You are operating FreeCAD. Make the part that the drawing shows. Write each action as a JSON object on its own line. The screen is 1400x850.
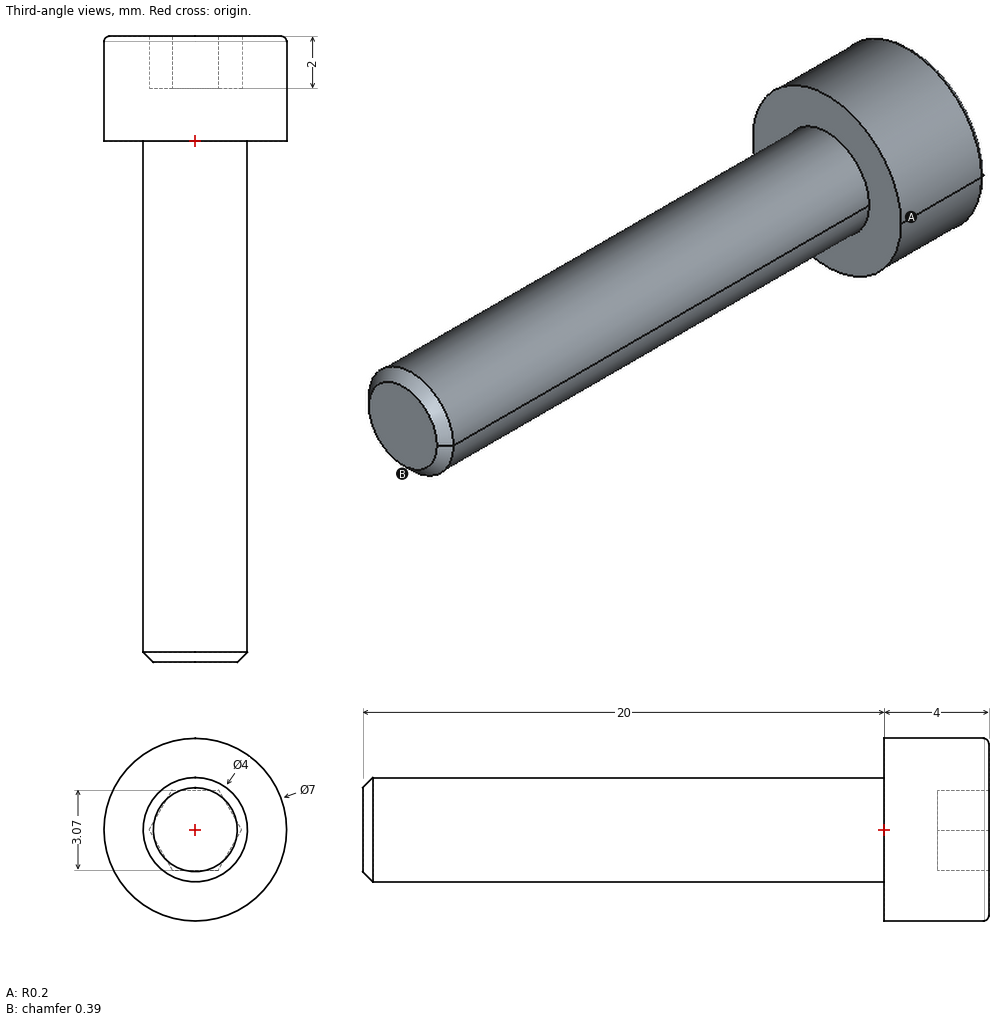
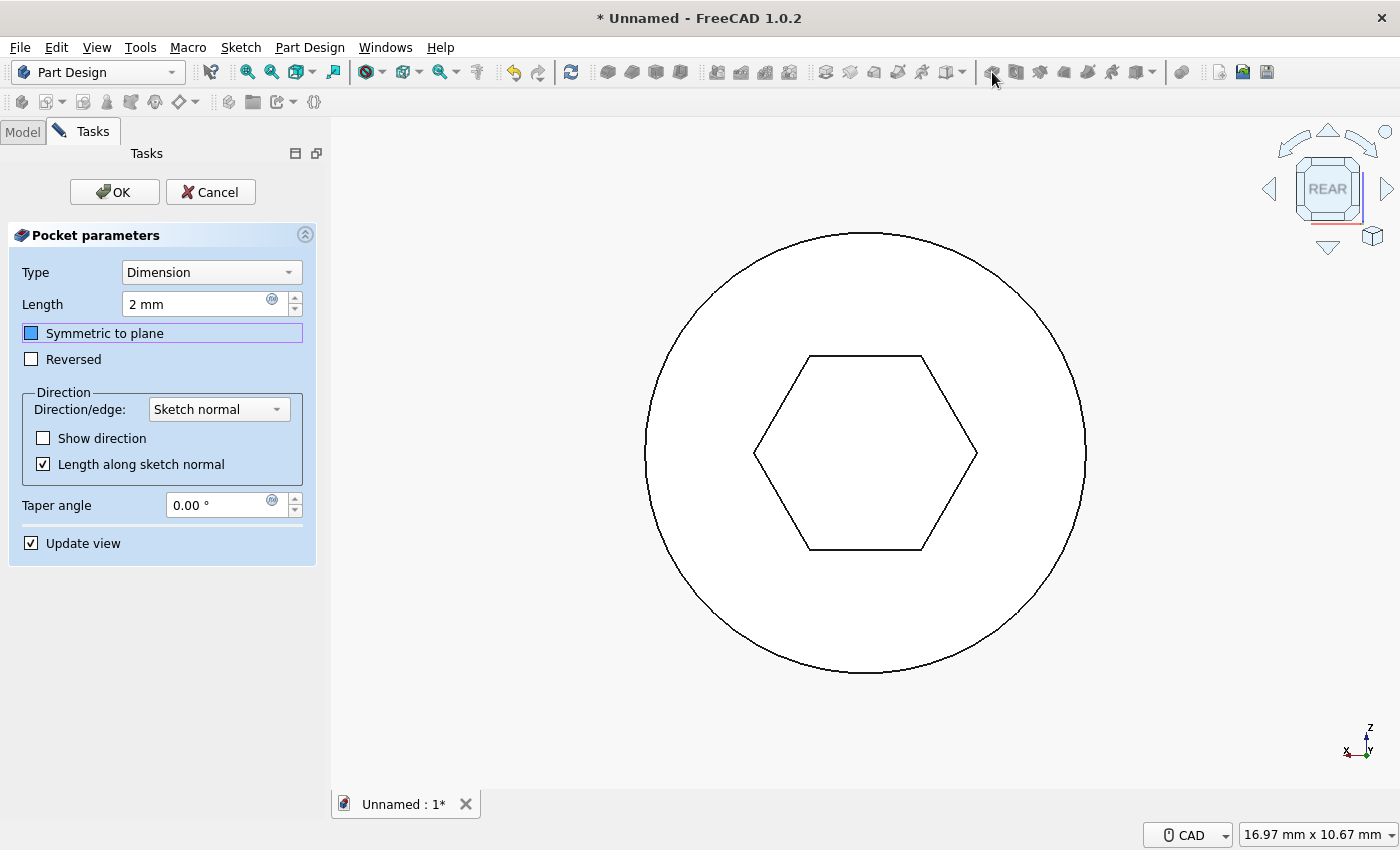
{"action": "left_click", "coordinate": [115, 192]}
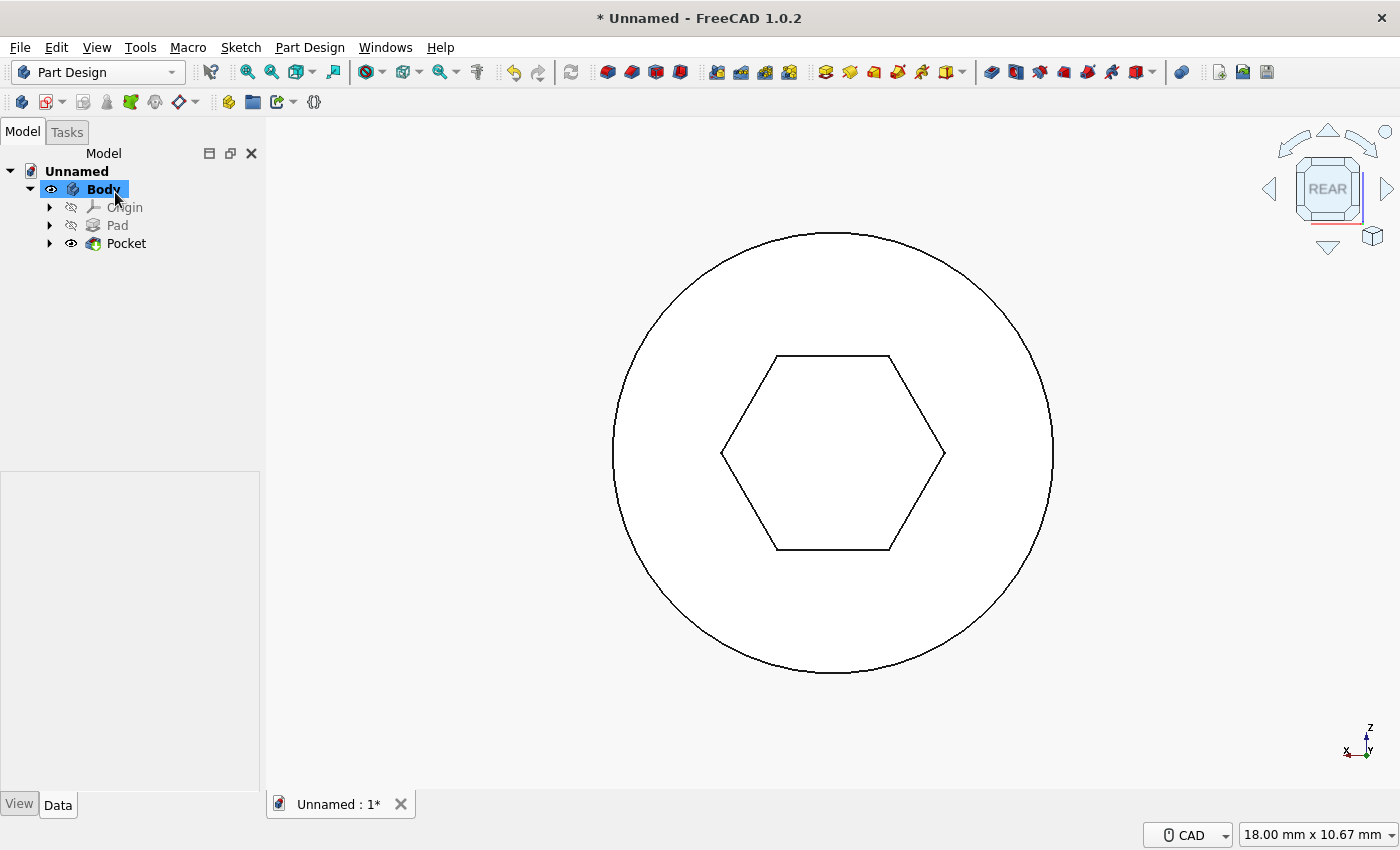
{"action": "left_click", "coordinate": [1053, 452]}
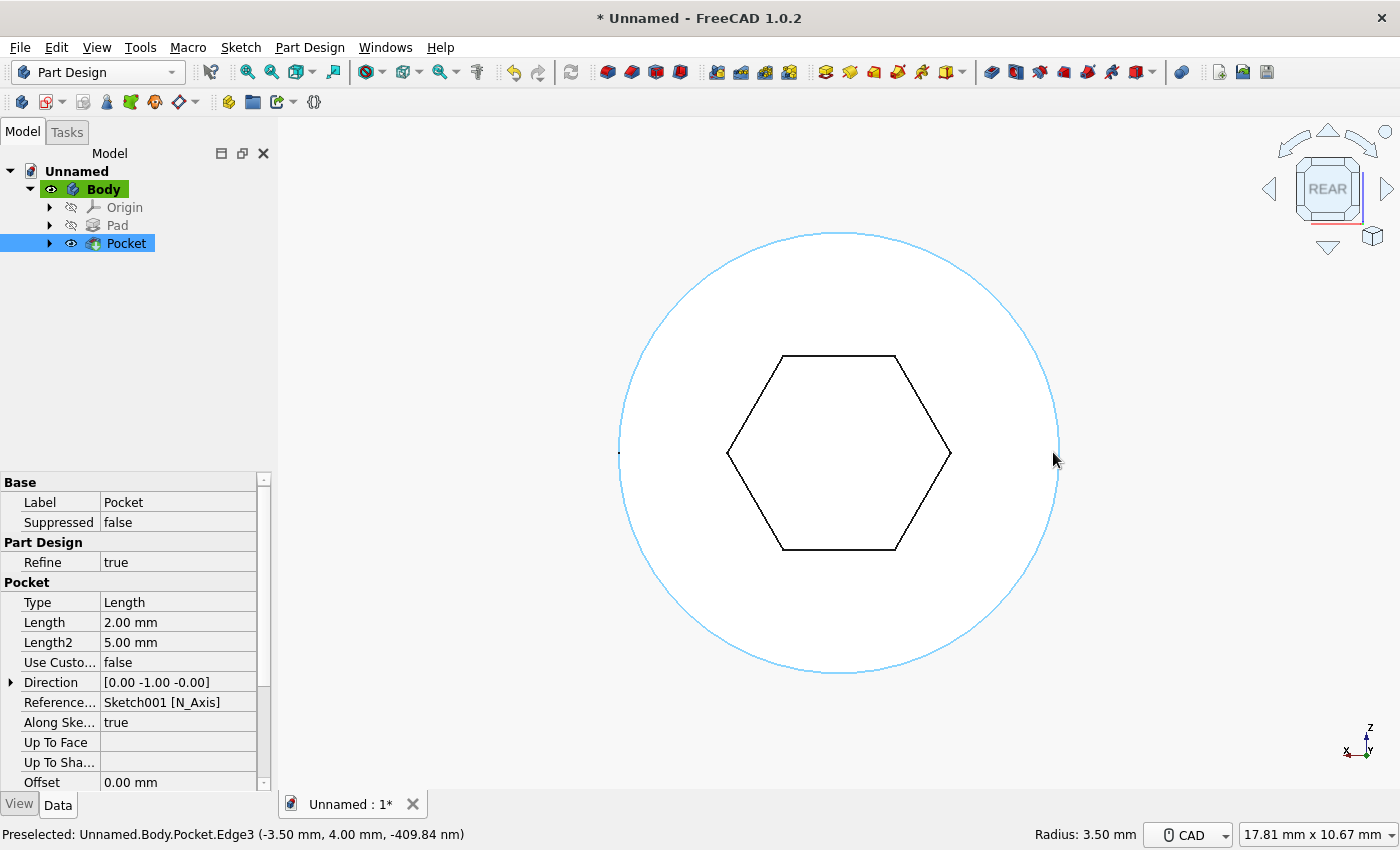
{"action": "left_click", "coordinate": [608, 72]}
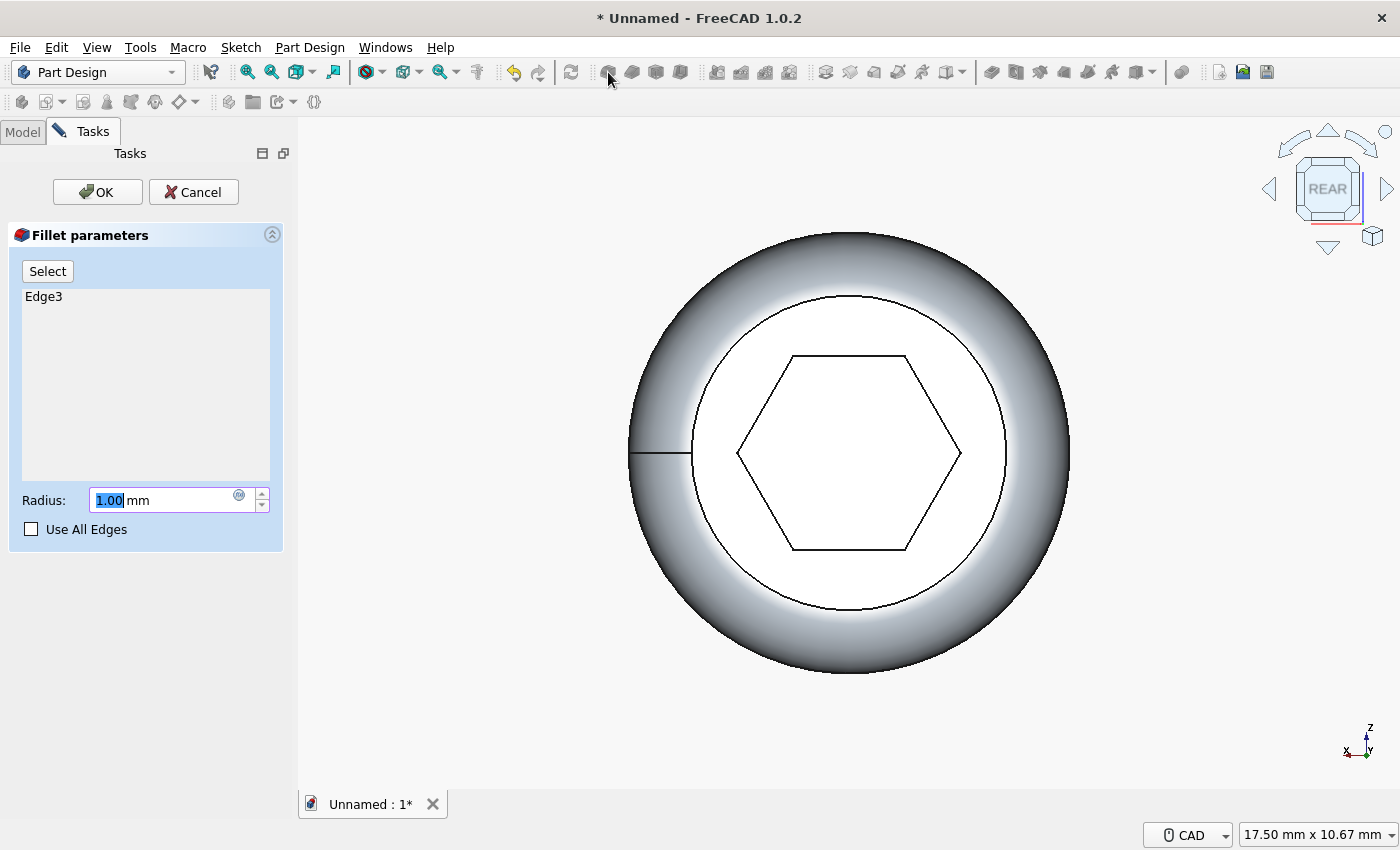
{"action": "type", "text": "0.2"}
{"action": "key", "text": "Tab"}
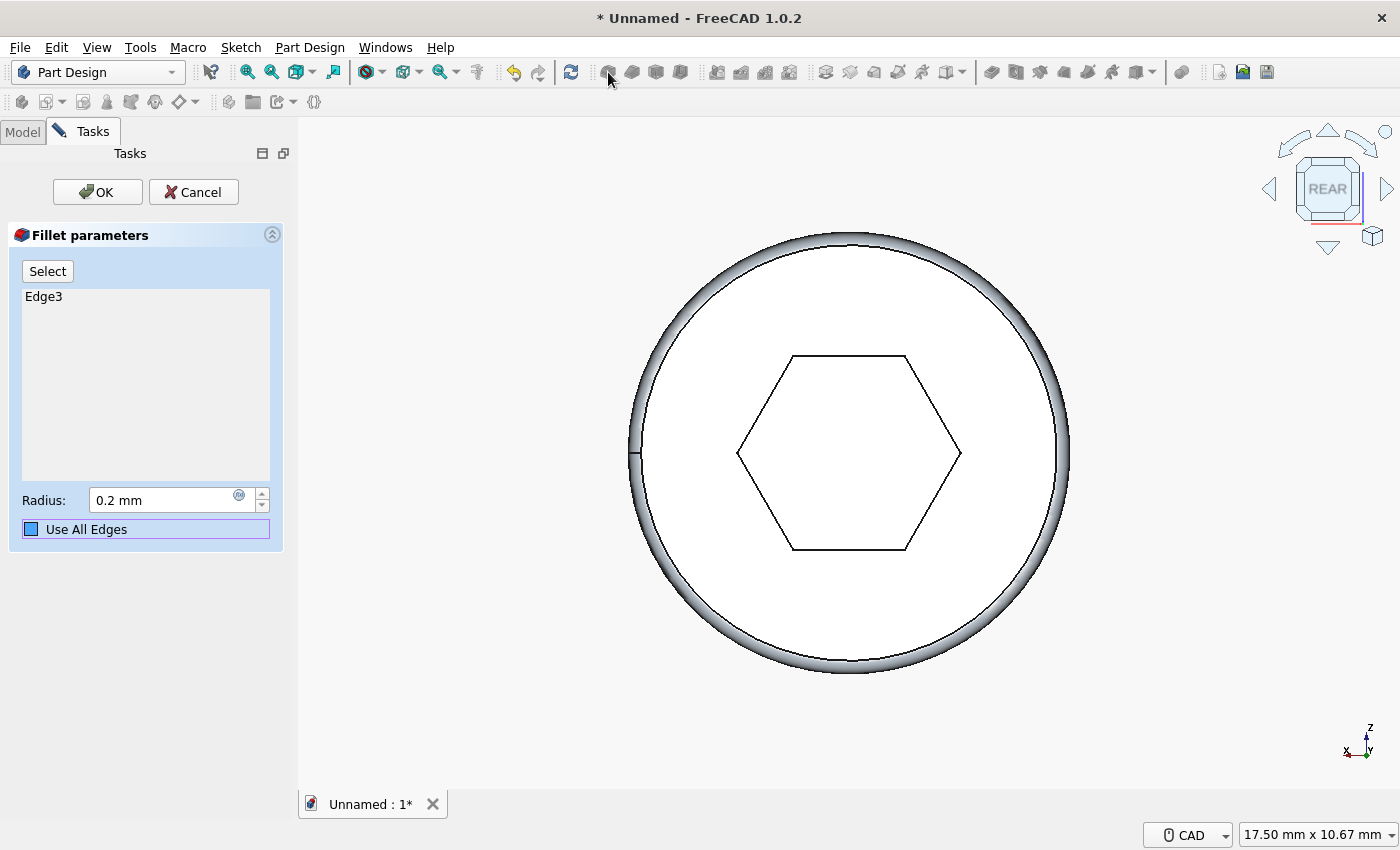
{"action": "left_click", "coordinate": [98, 192]}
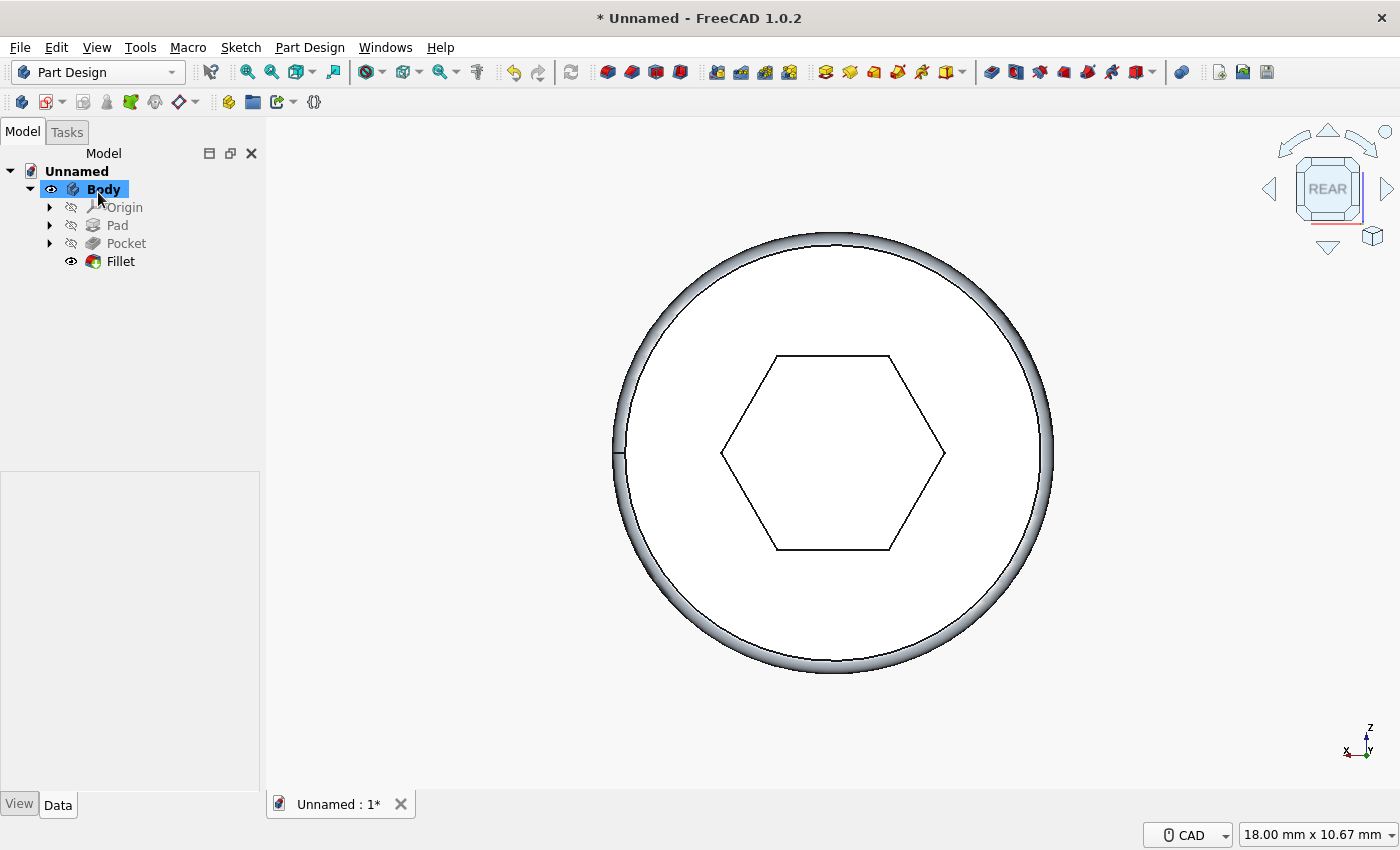
{"action": "left_click", "coordinate": [46, 102]}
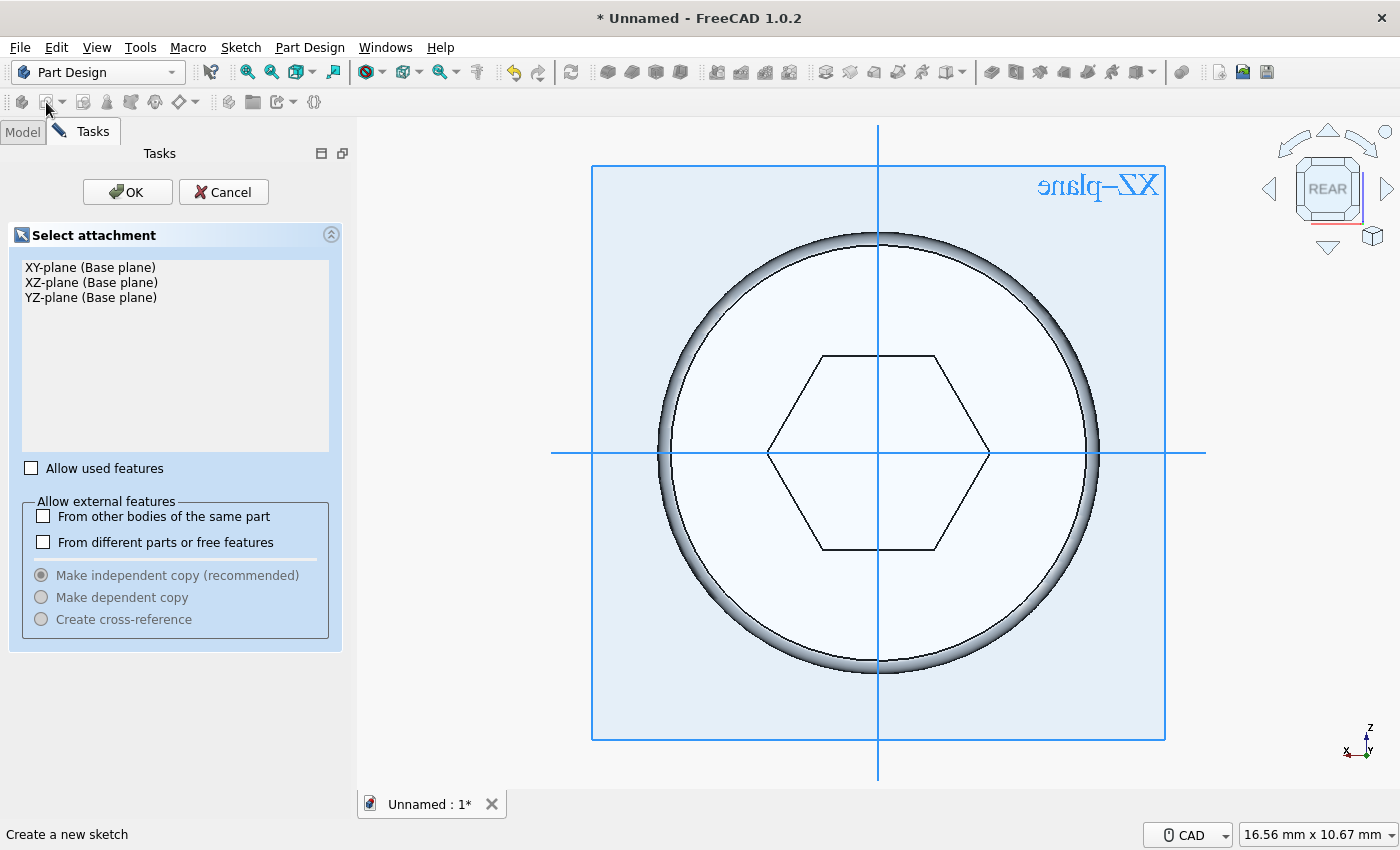
{"action": "left_click", "coordinate": [82, 282]}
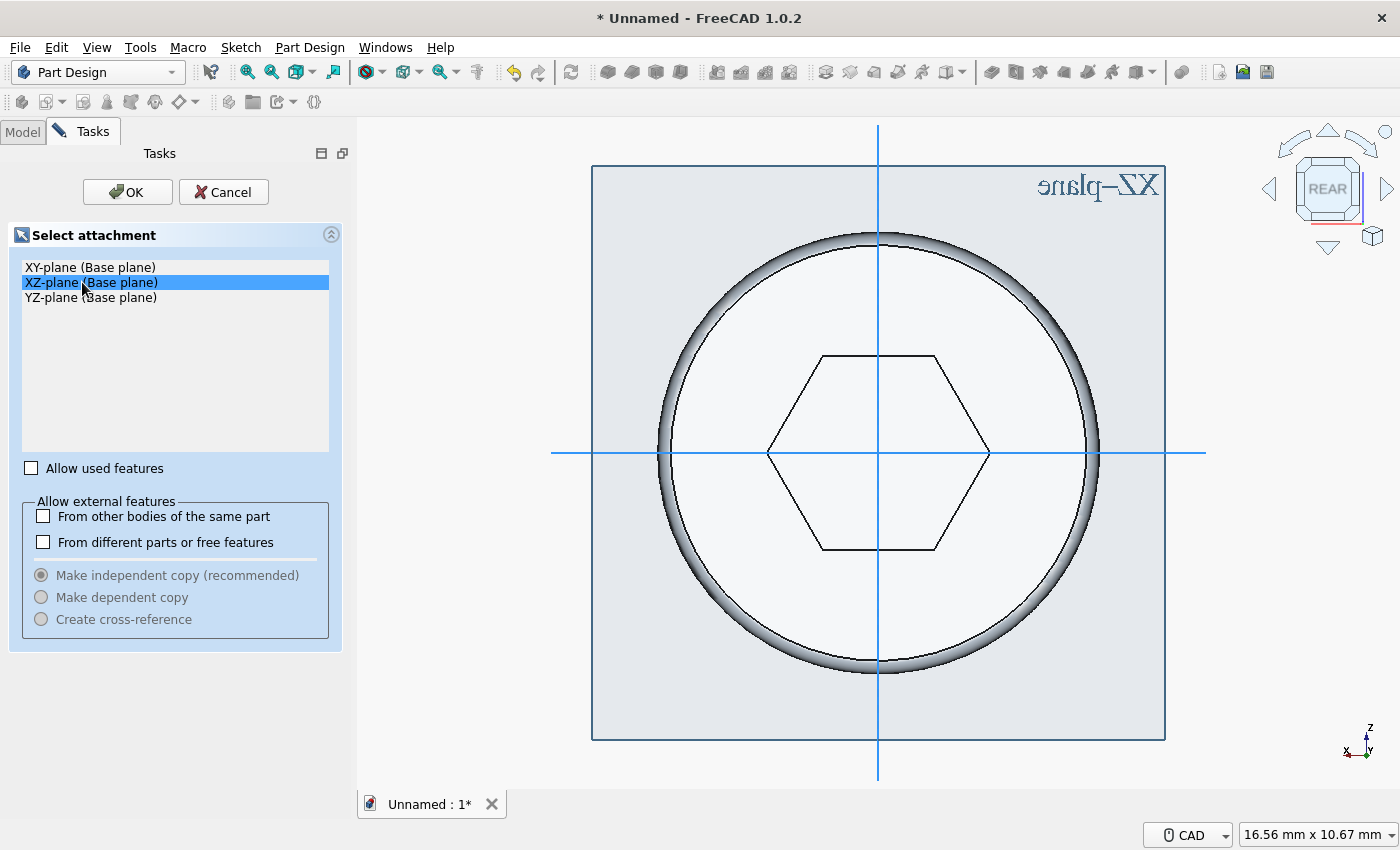
{"action": "left_click", "coordinate": [128, 192]}